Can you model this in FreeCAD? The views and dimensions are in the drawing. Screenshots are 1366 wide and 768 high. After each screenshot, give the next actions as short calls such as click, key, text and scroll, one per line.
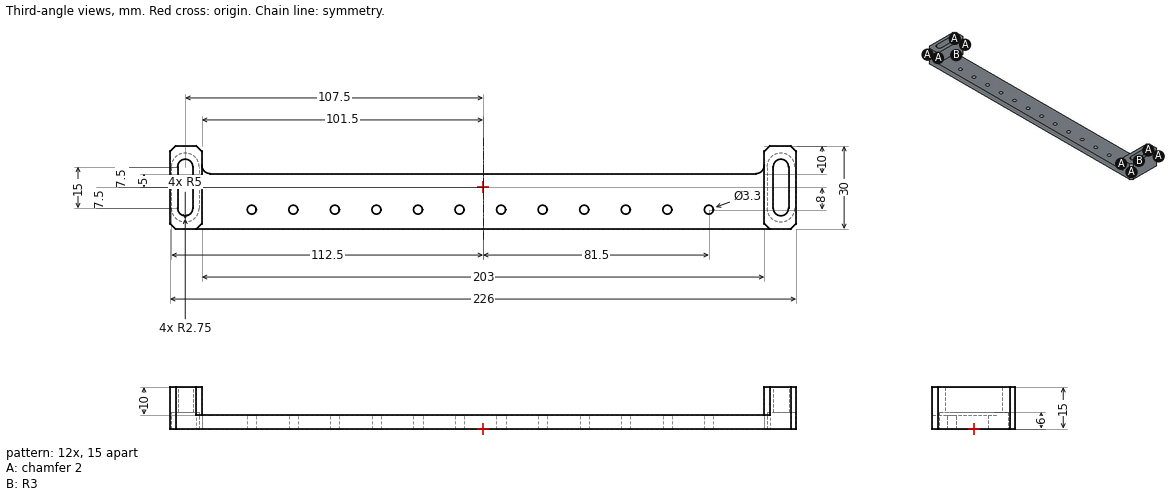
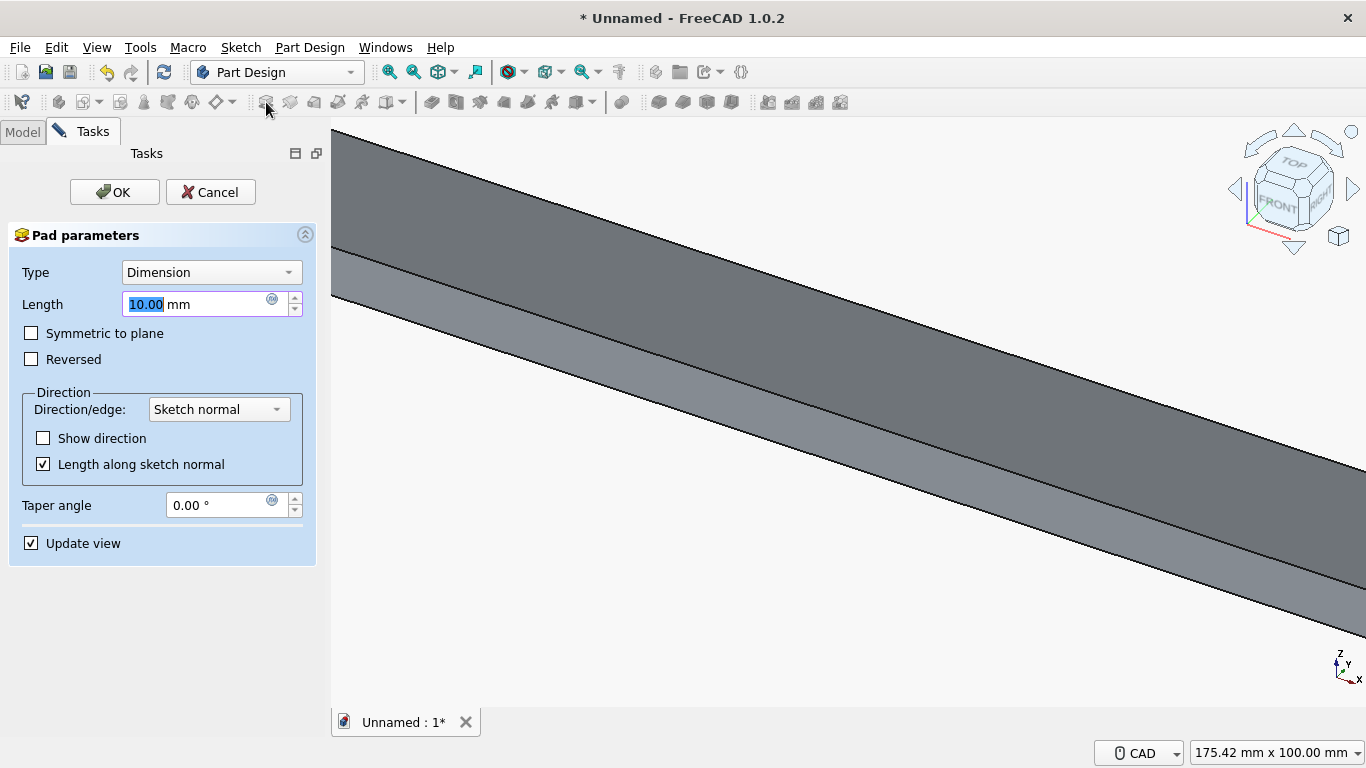
text(15)
key(Tab)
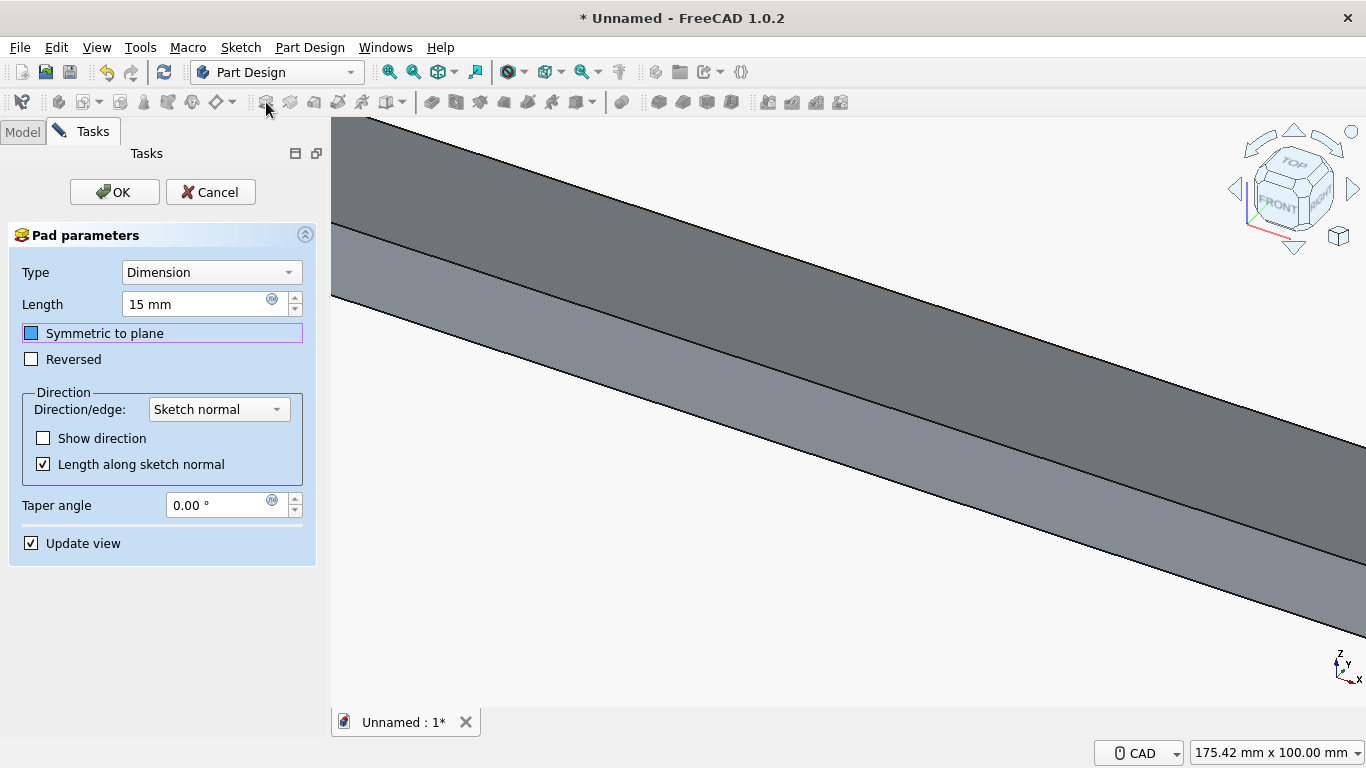
click(115, 192)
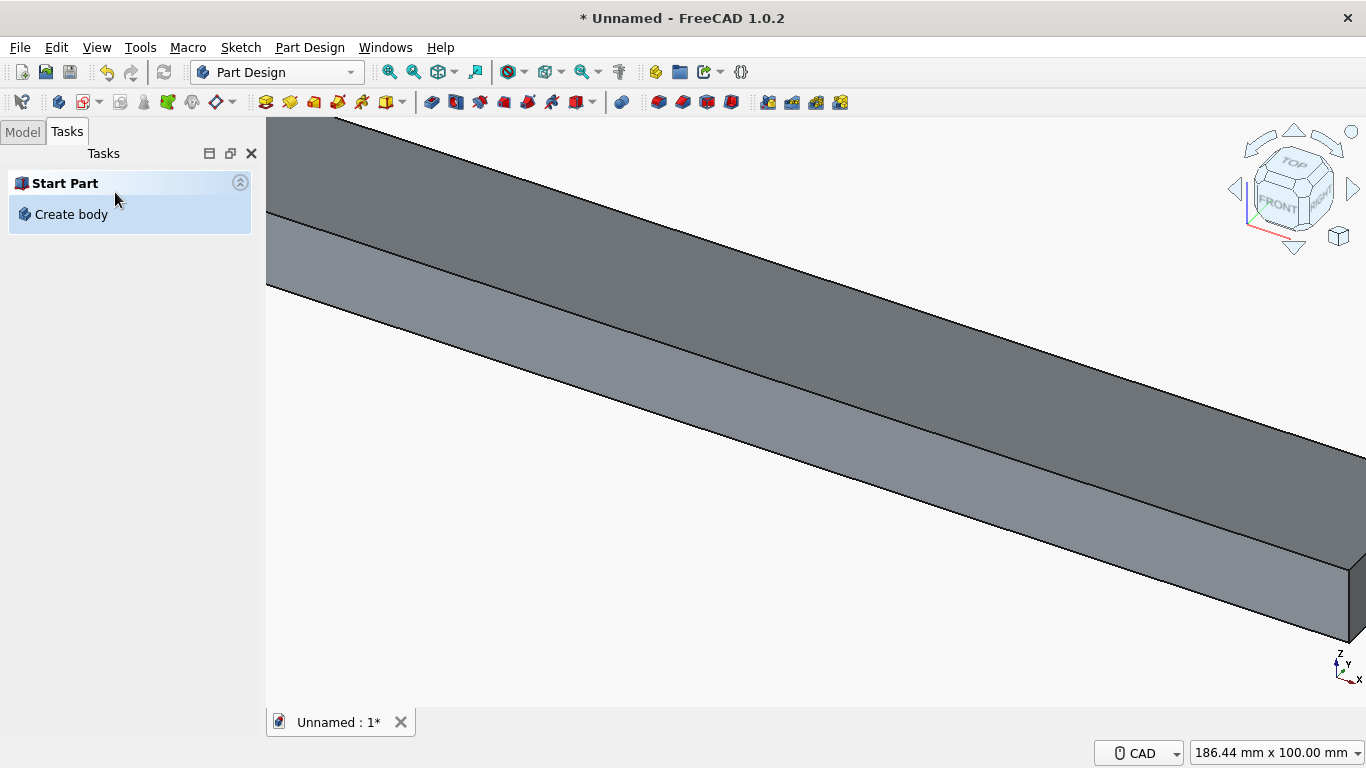
click(390, 72)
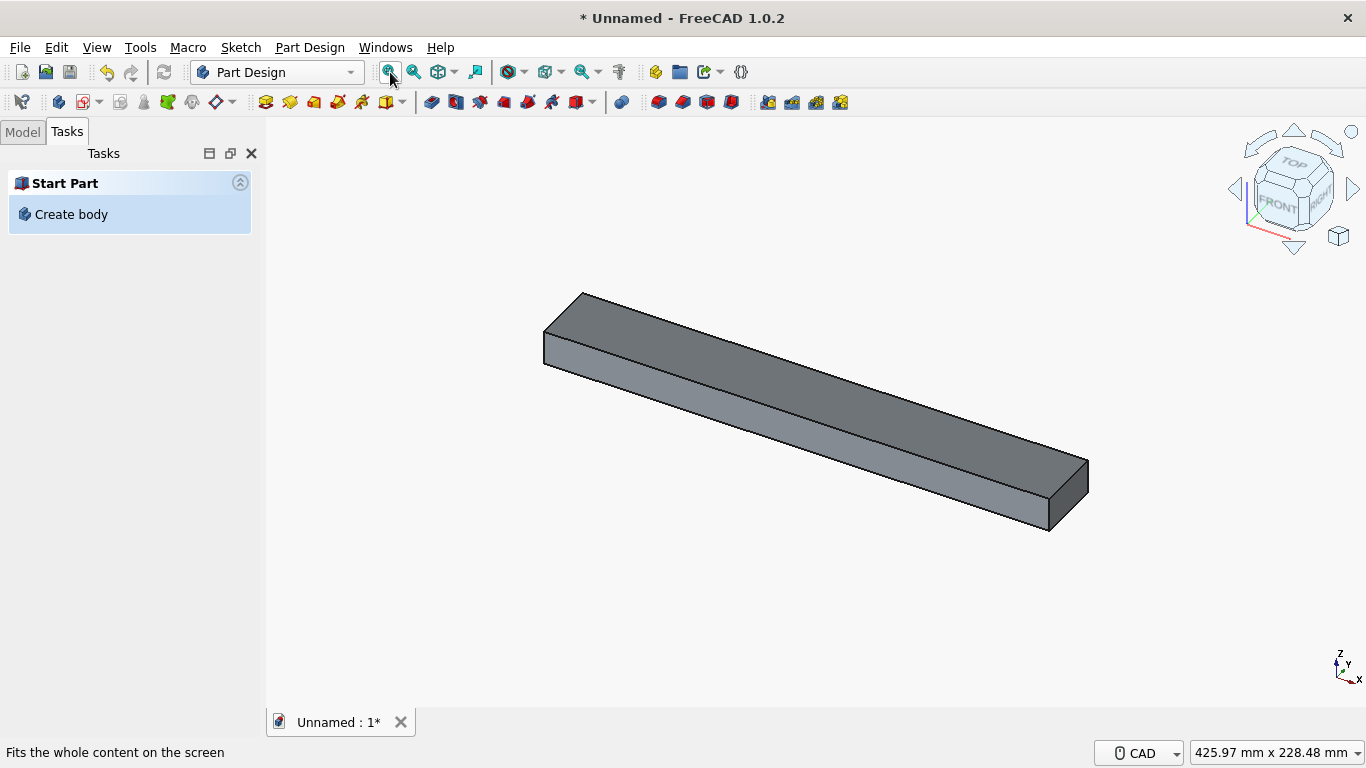
click(1033, 467)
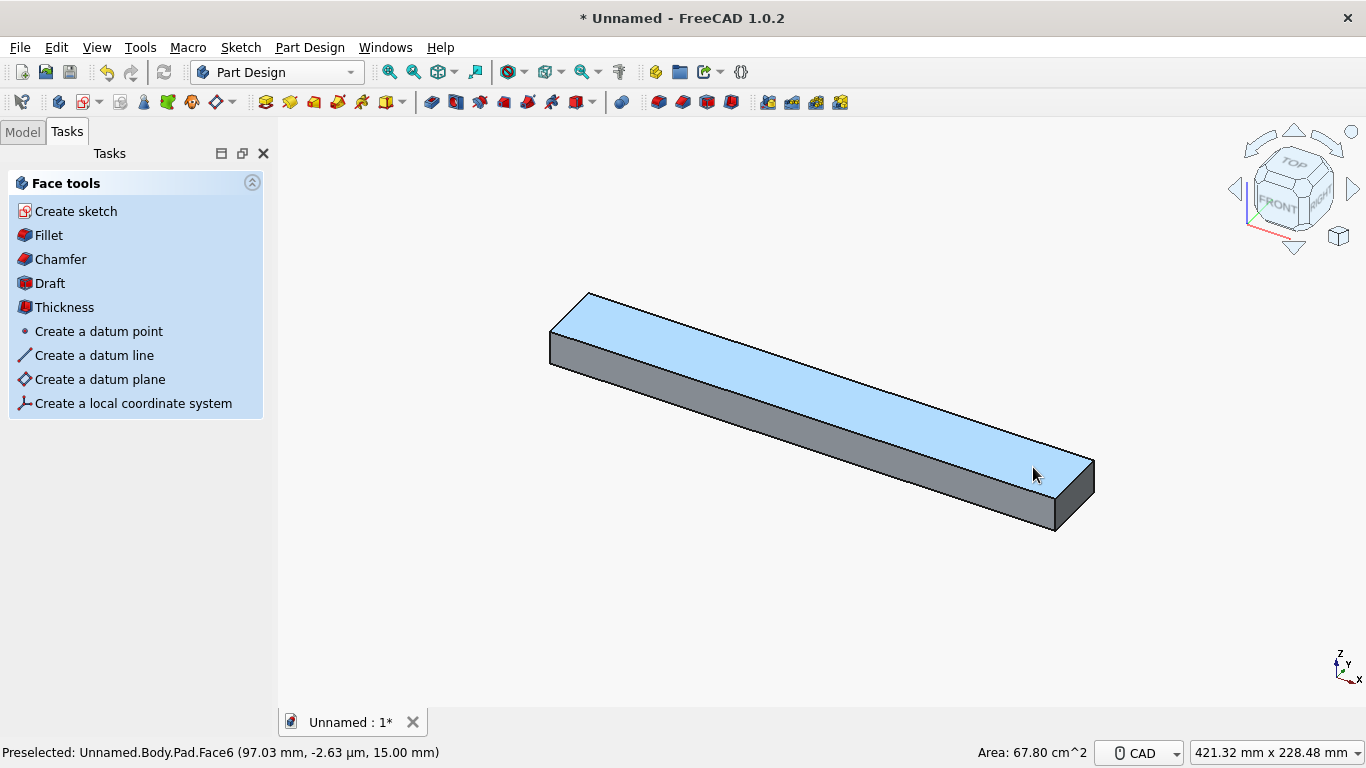
click(84, 102)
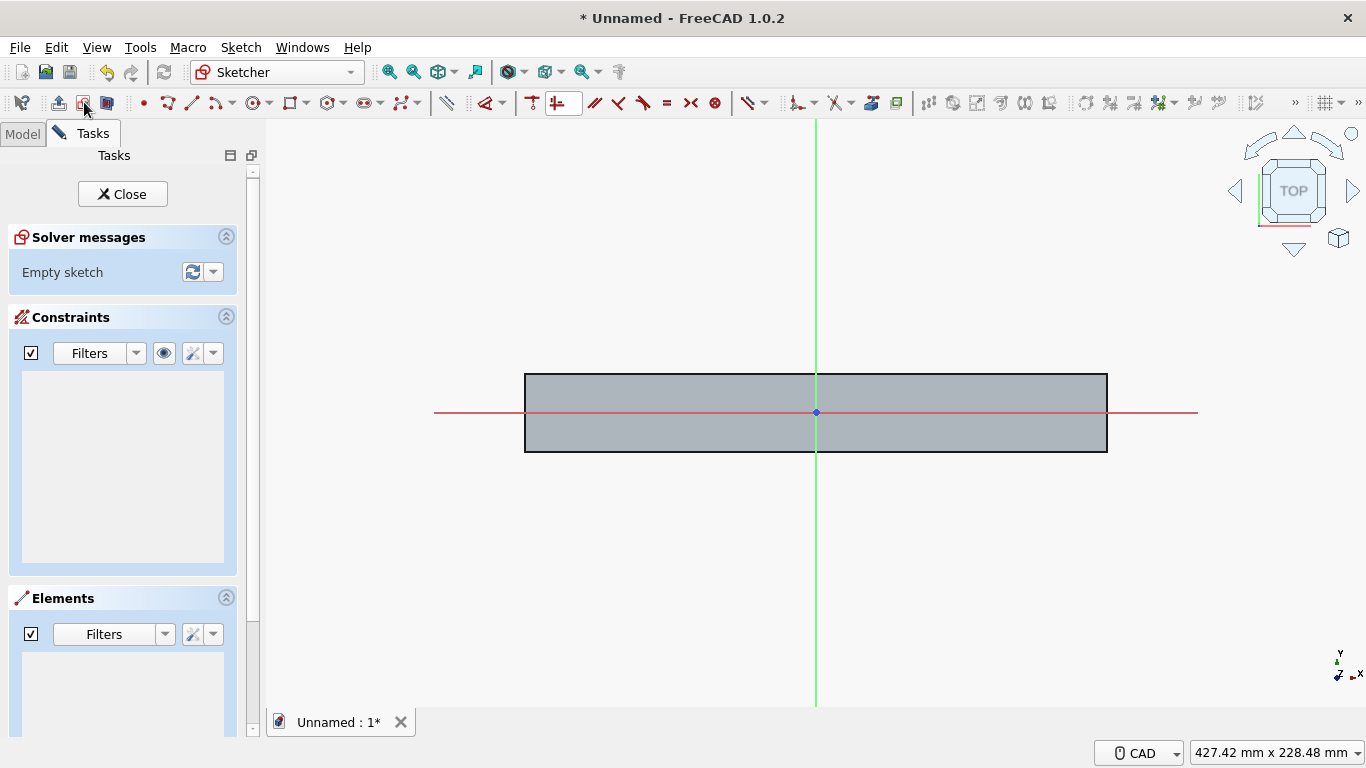
key(g)
key(v)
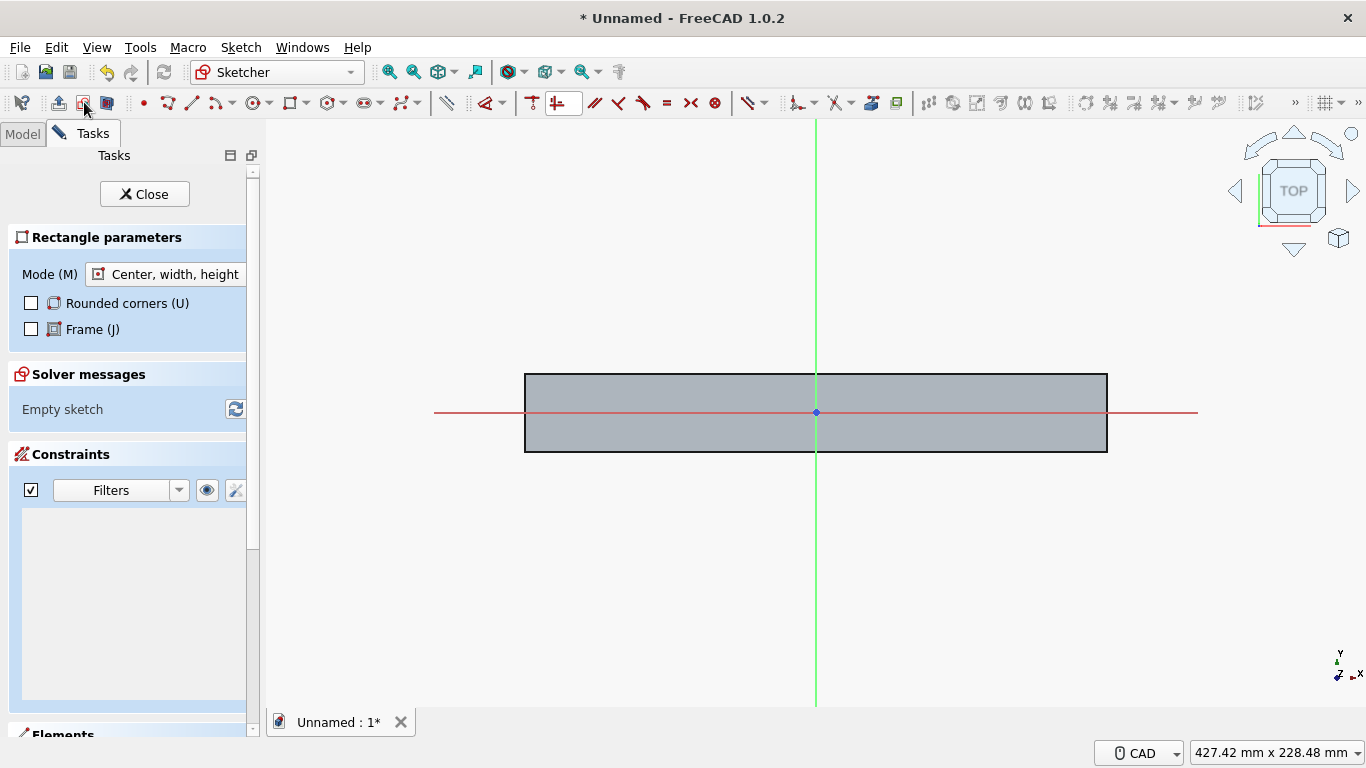
click(816, 413)
move(1077, 374)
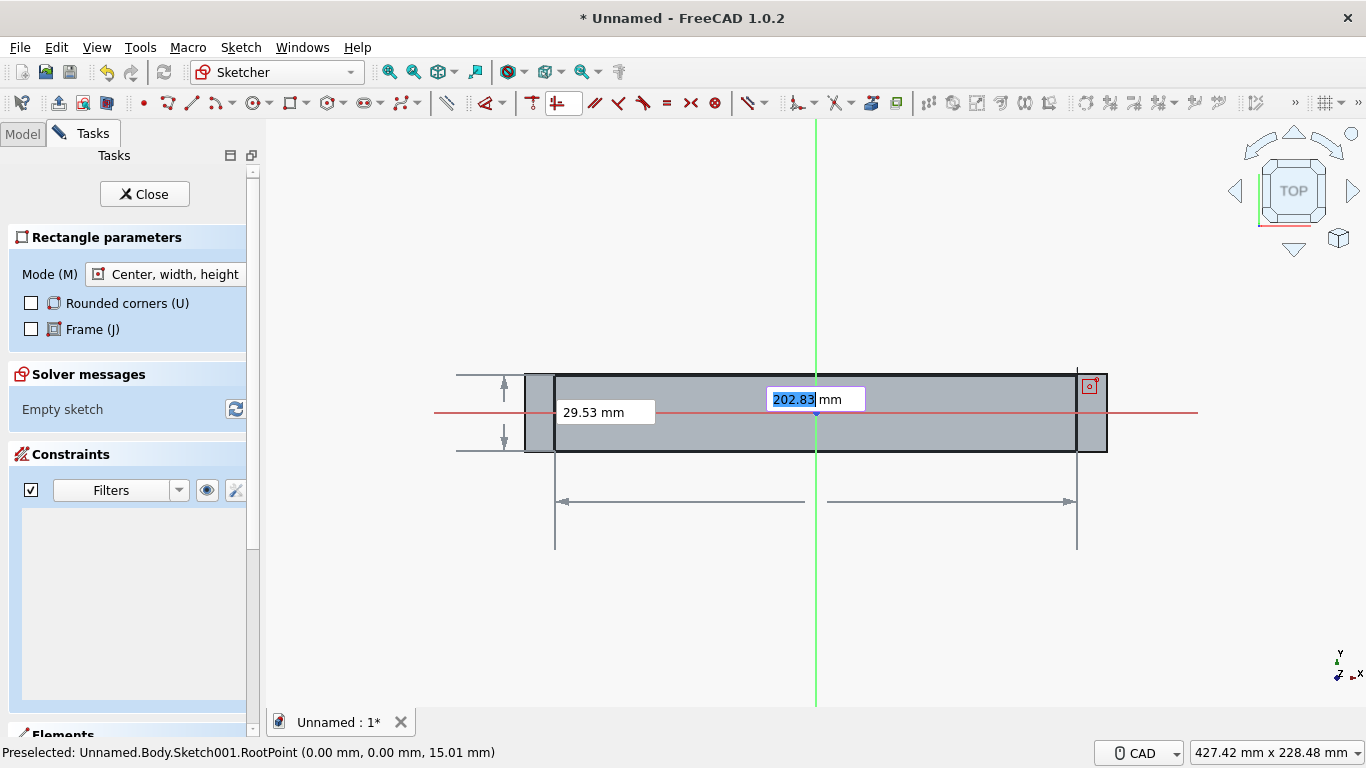
text(203)
key(Tab)
text(30)
key(Return)
key(Escape)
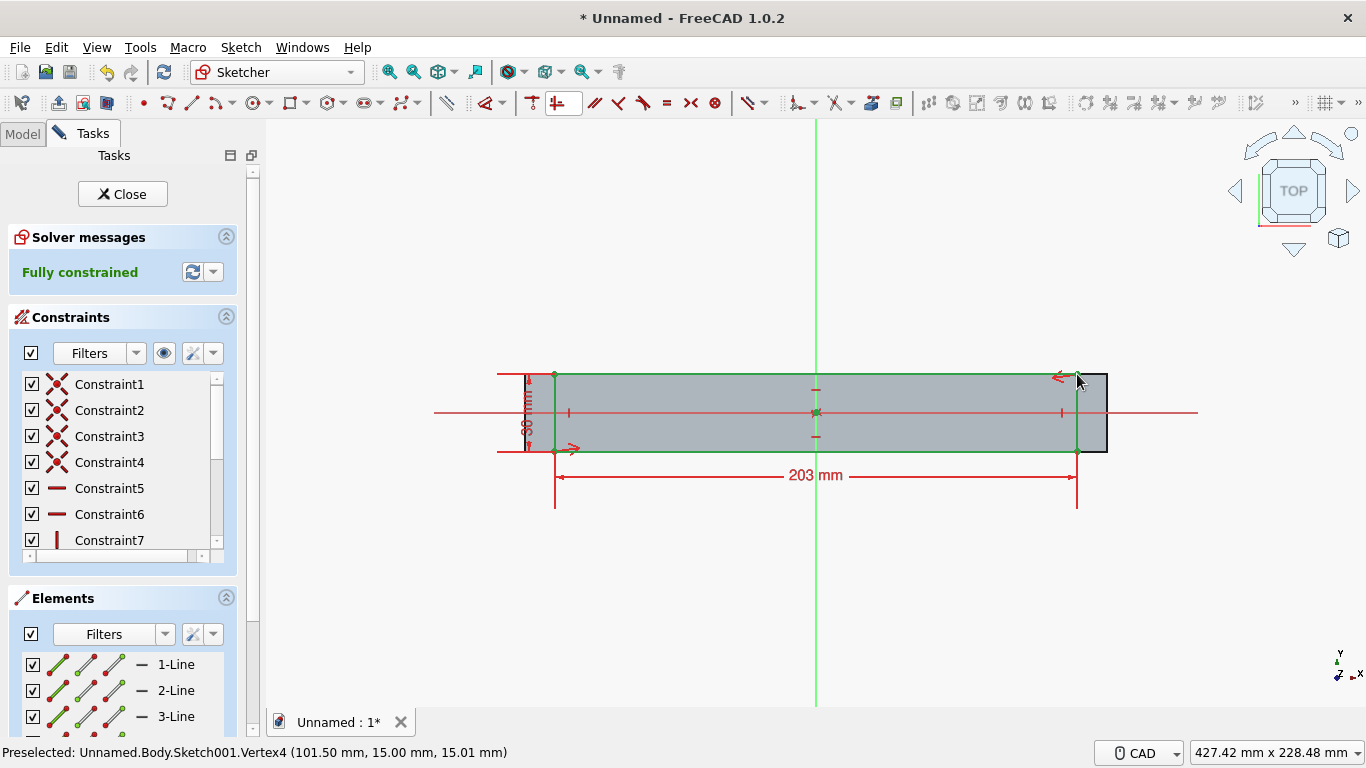
click(123, 194)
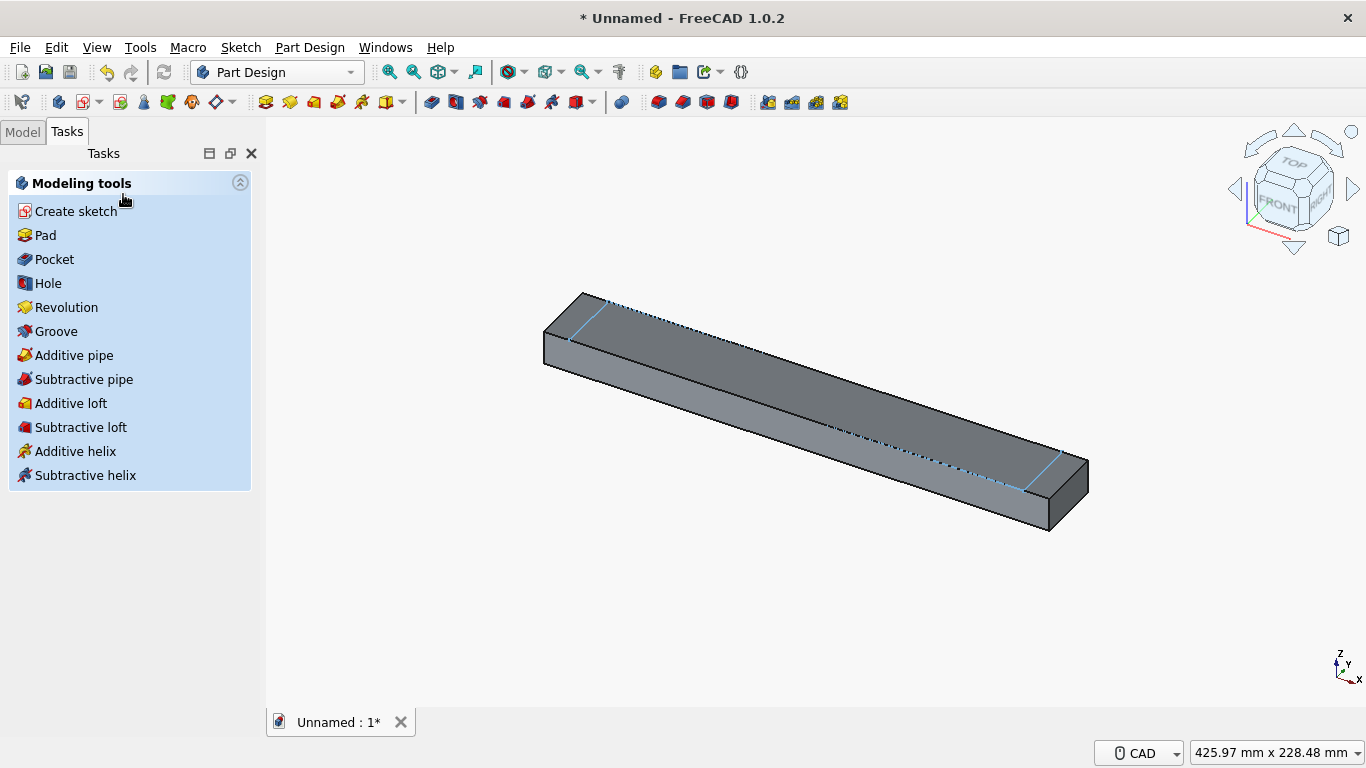
click(432, 102)